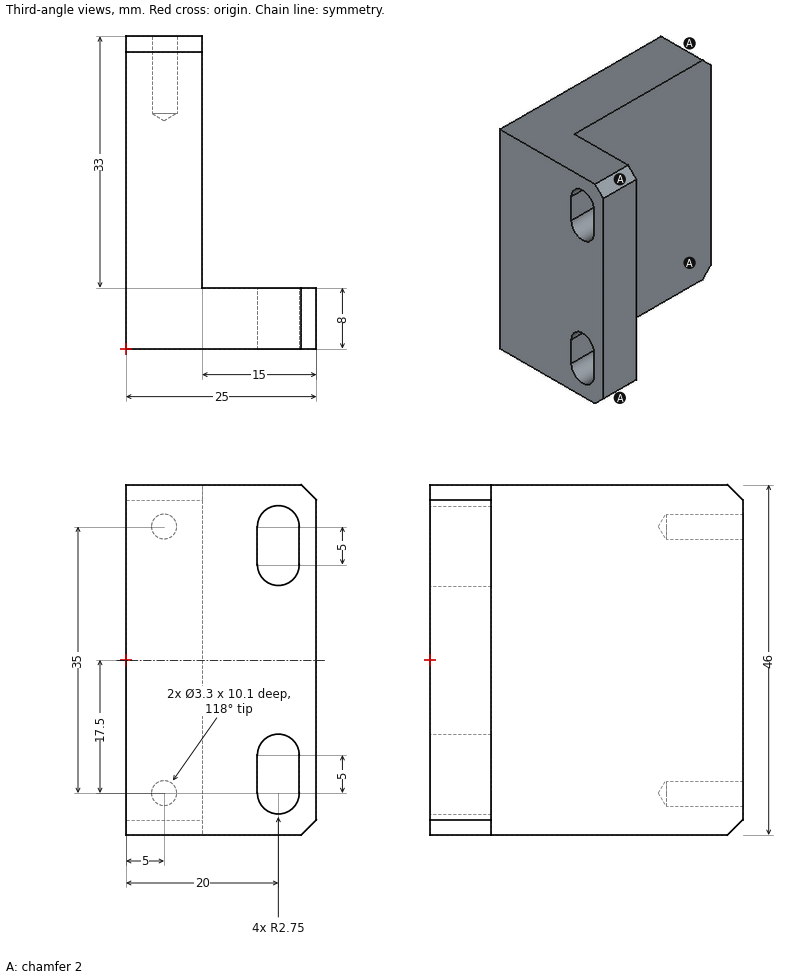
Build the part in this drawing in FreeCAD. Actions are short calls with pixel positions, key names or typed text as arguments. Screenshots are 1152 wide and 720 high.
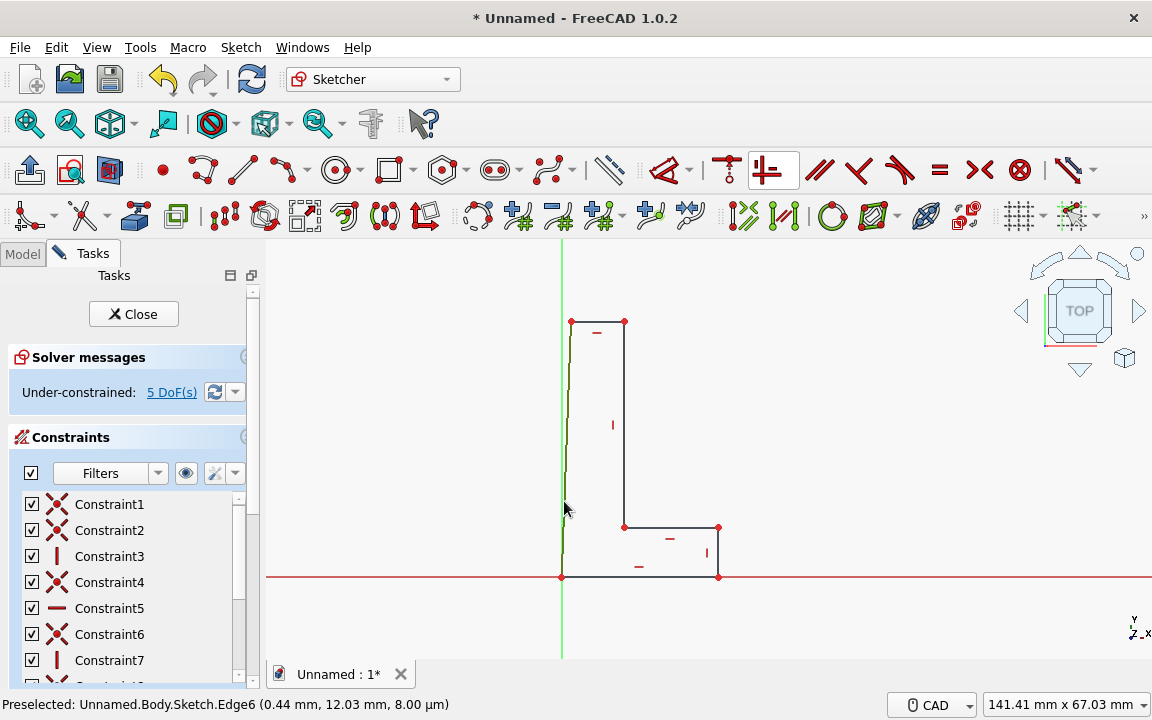
click(794, 170)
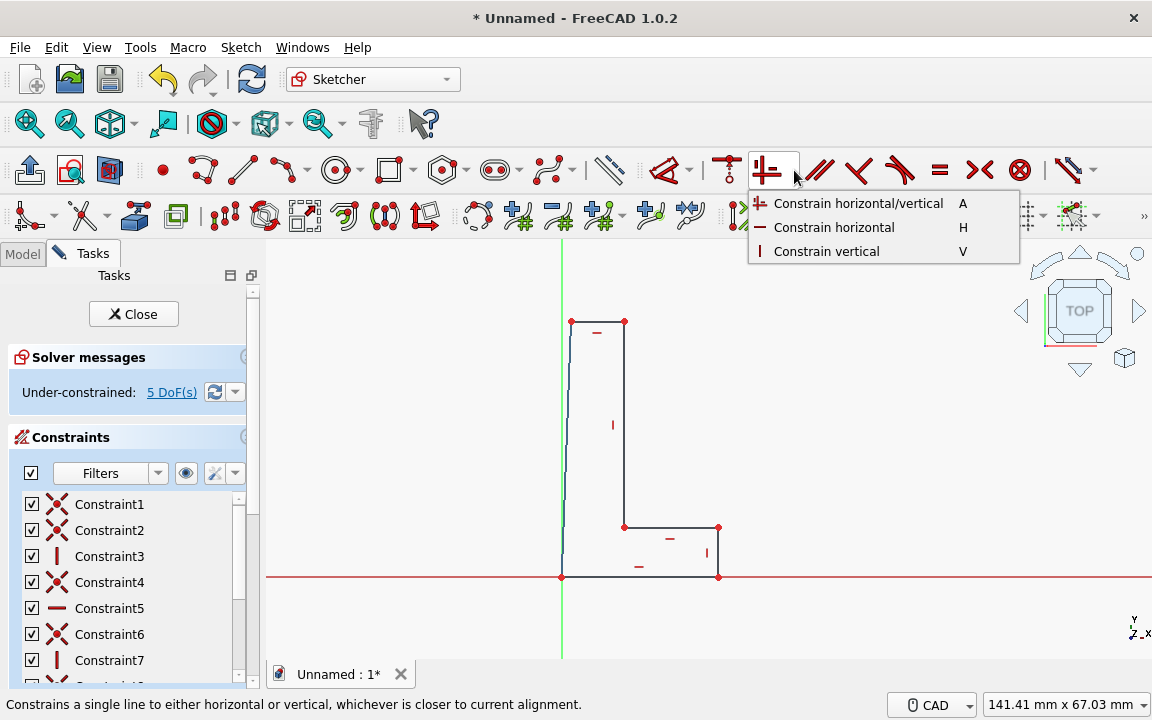
click(884, 251)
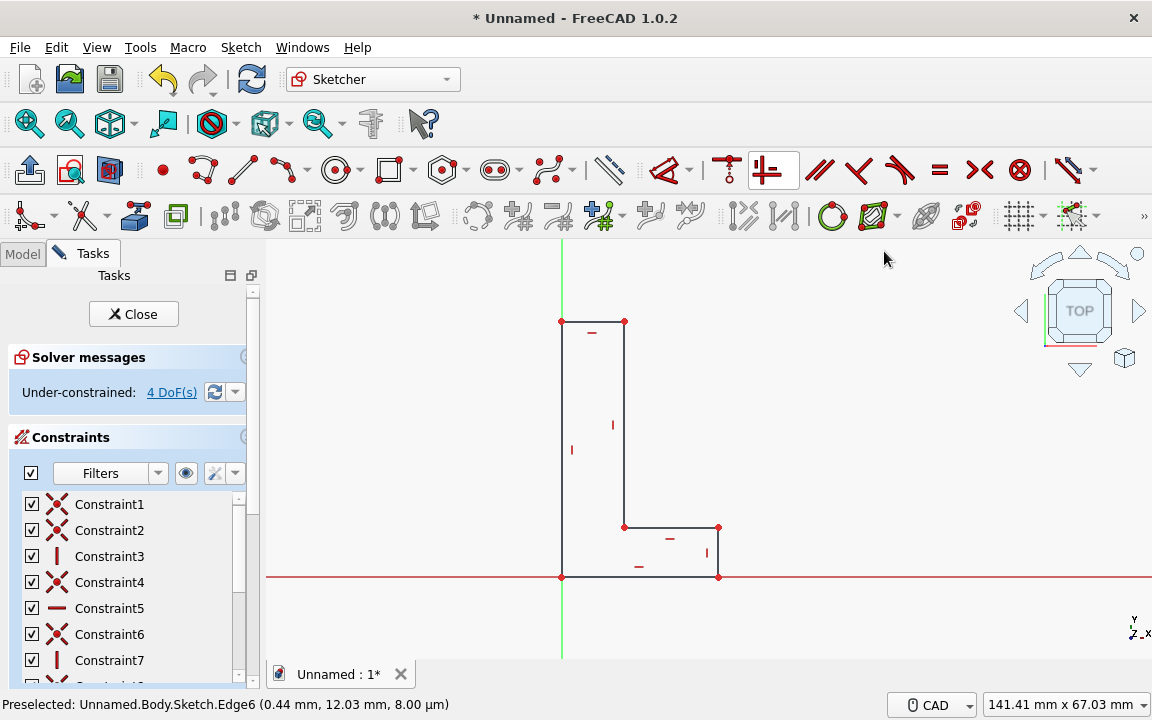
click(718, 563)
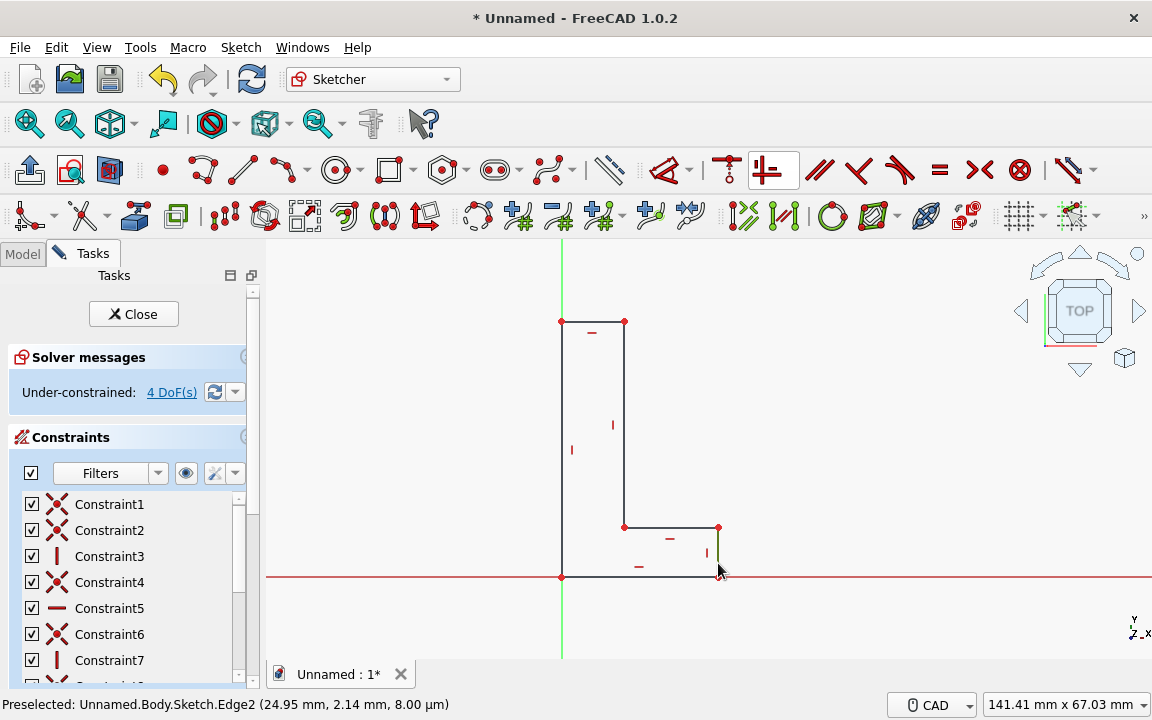
key(i)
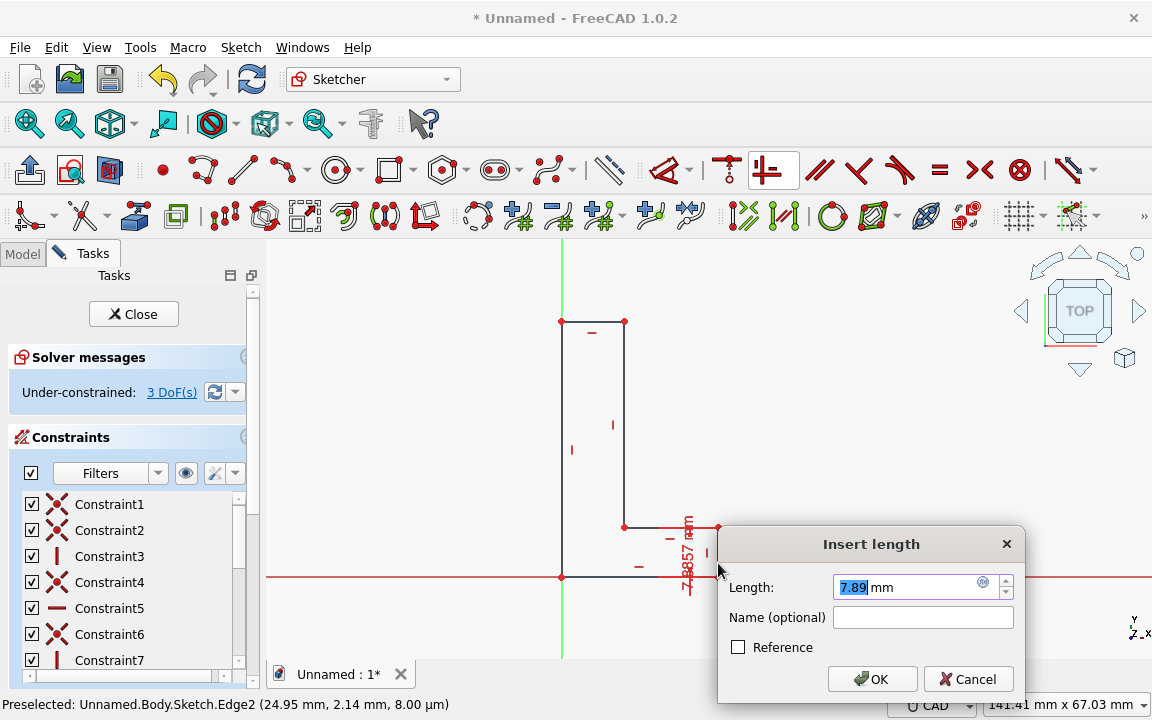
text(8)
key(Return)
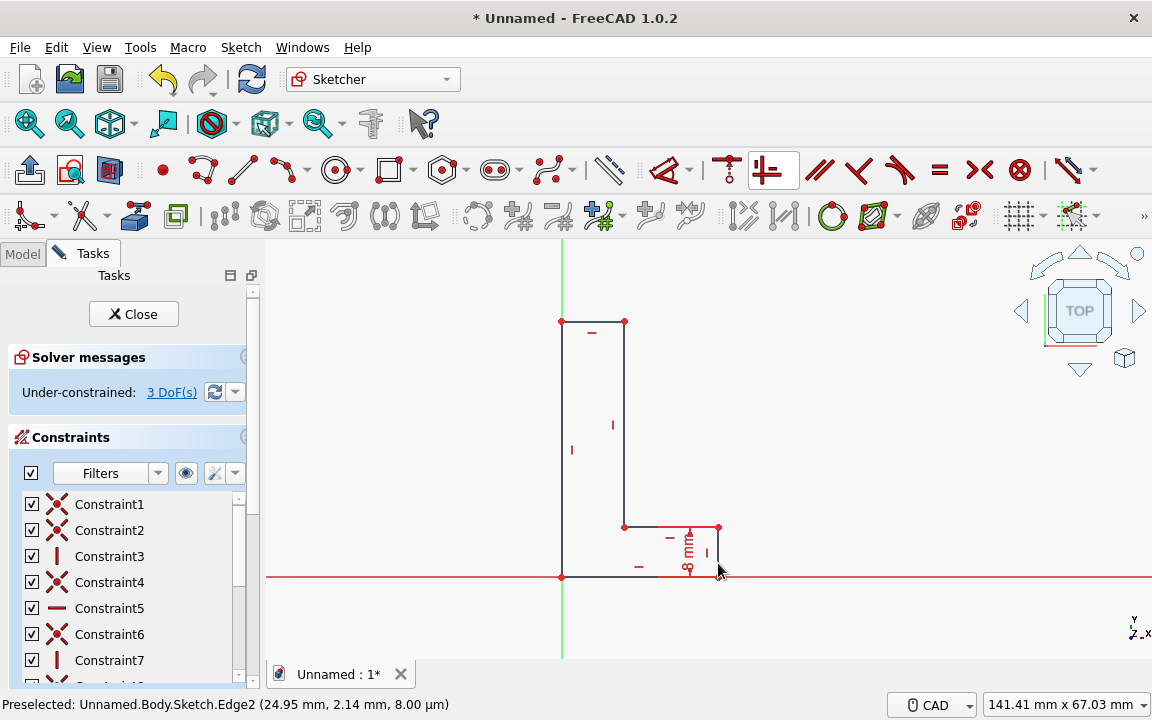
click(609, 577)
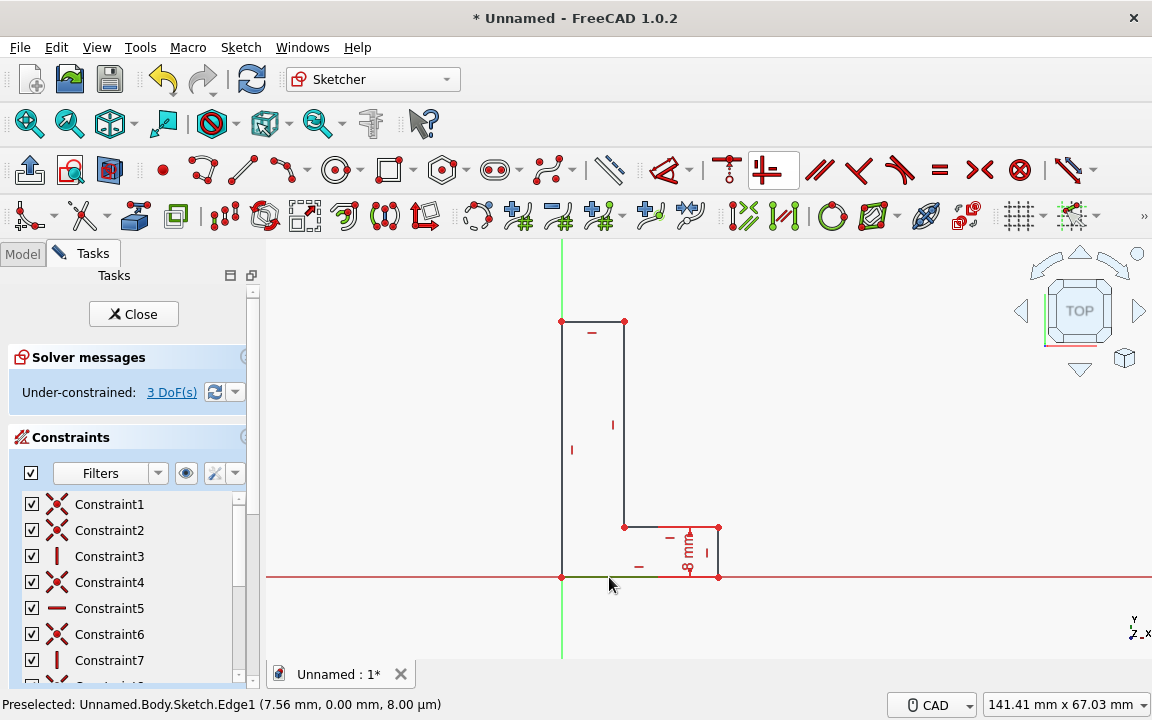
click(692, 170)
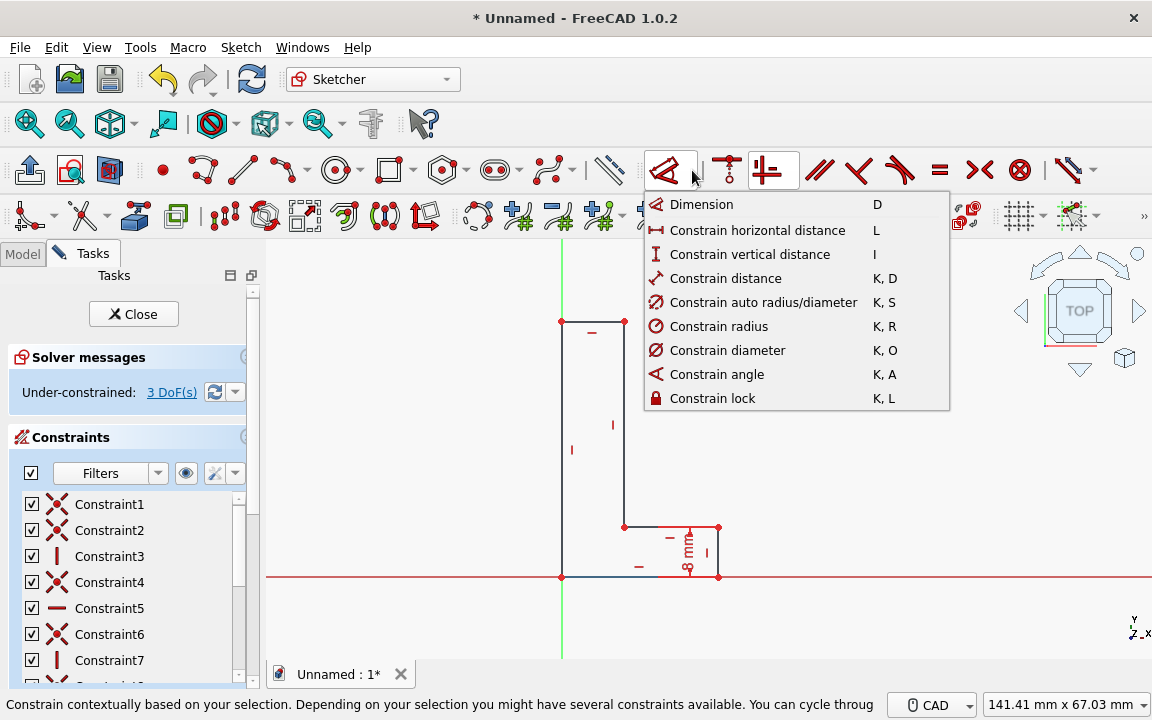
click(797, 230)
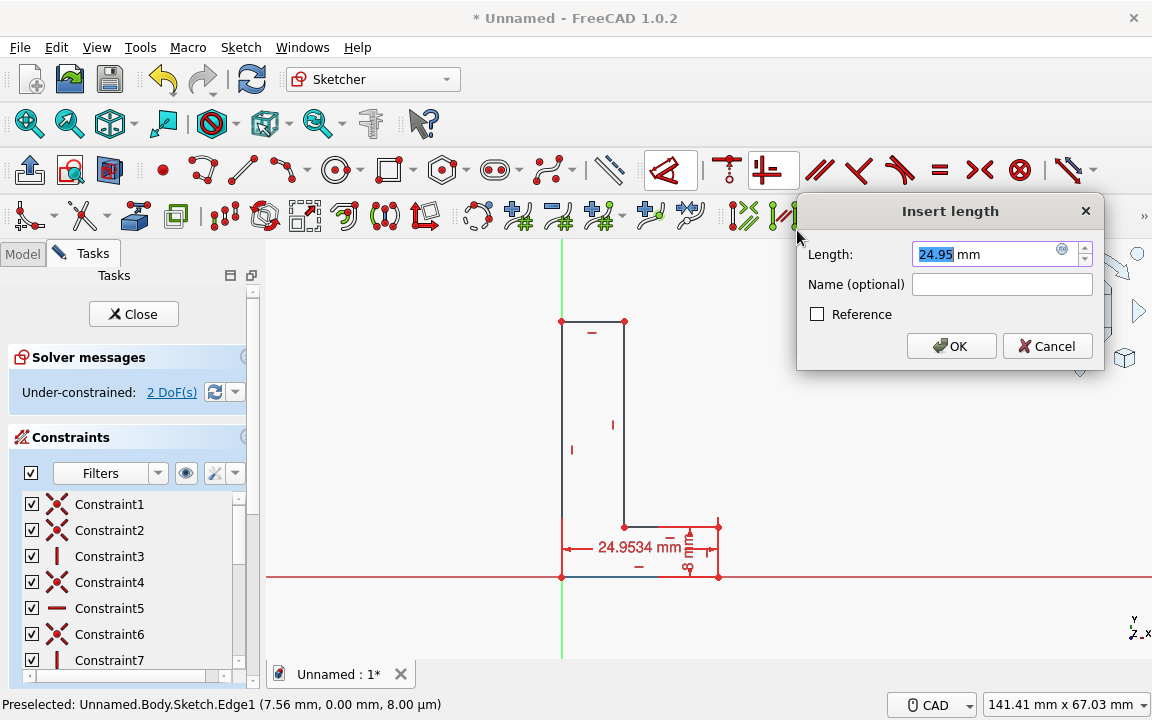
text(25)
key(Return)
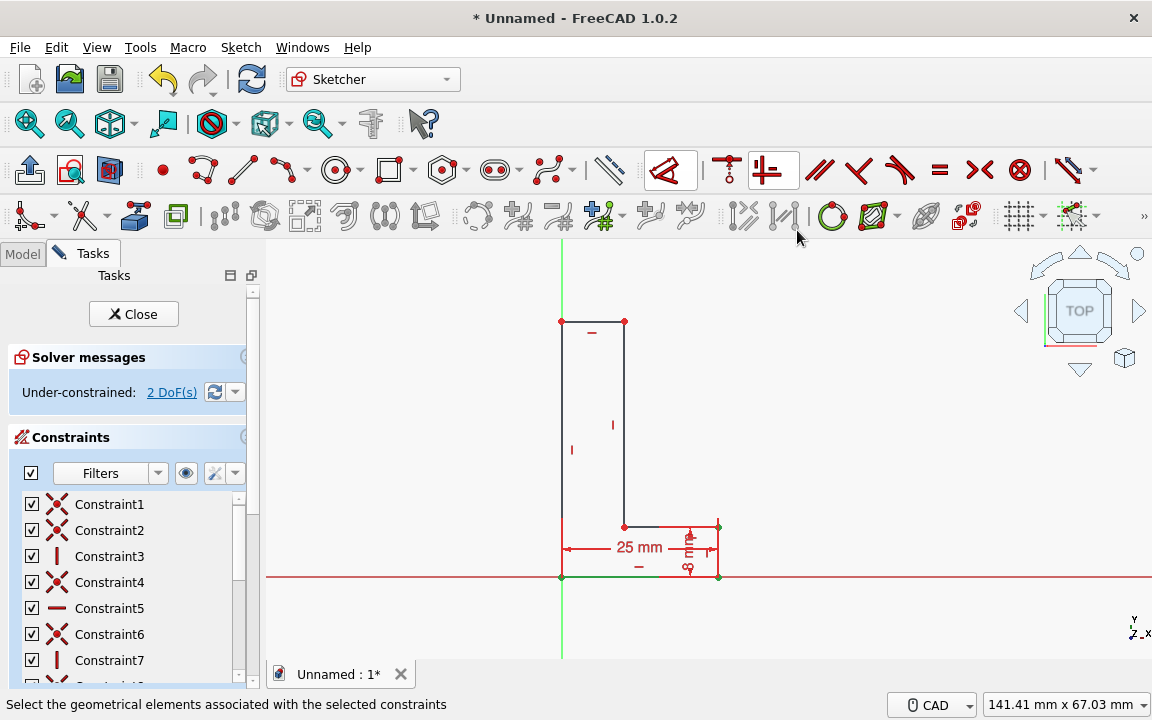
click(690, 527)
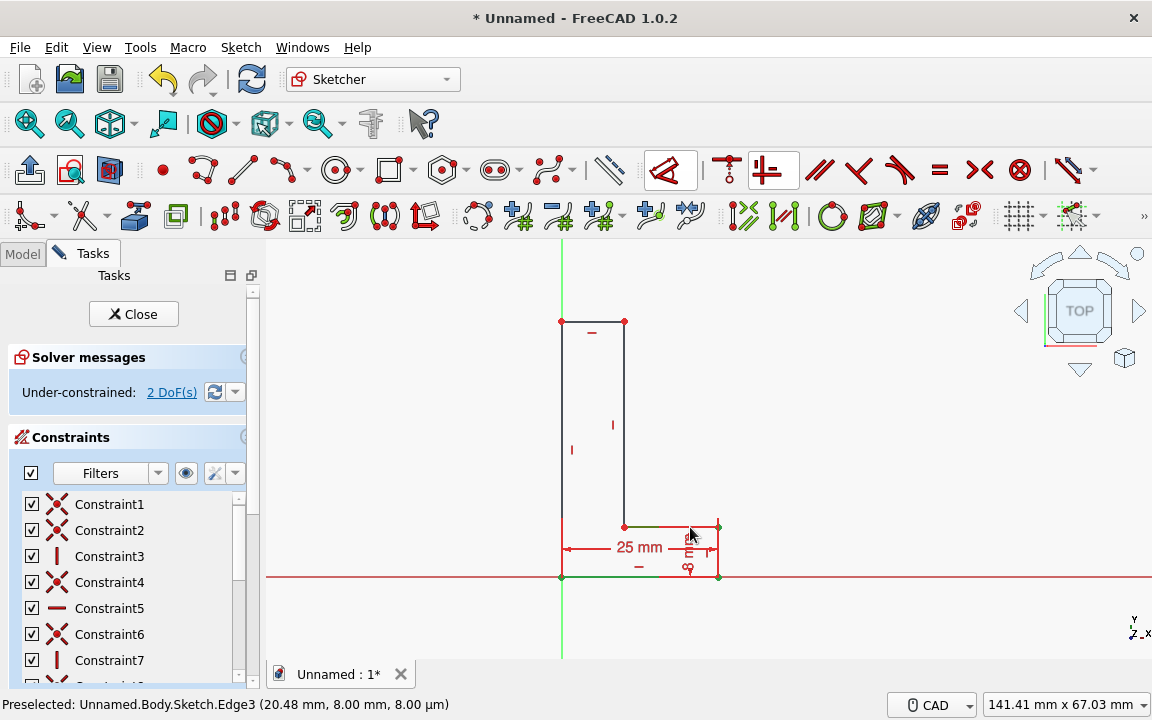
key(l)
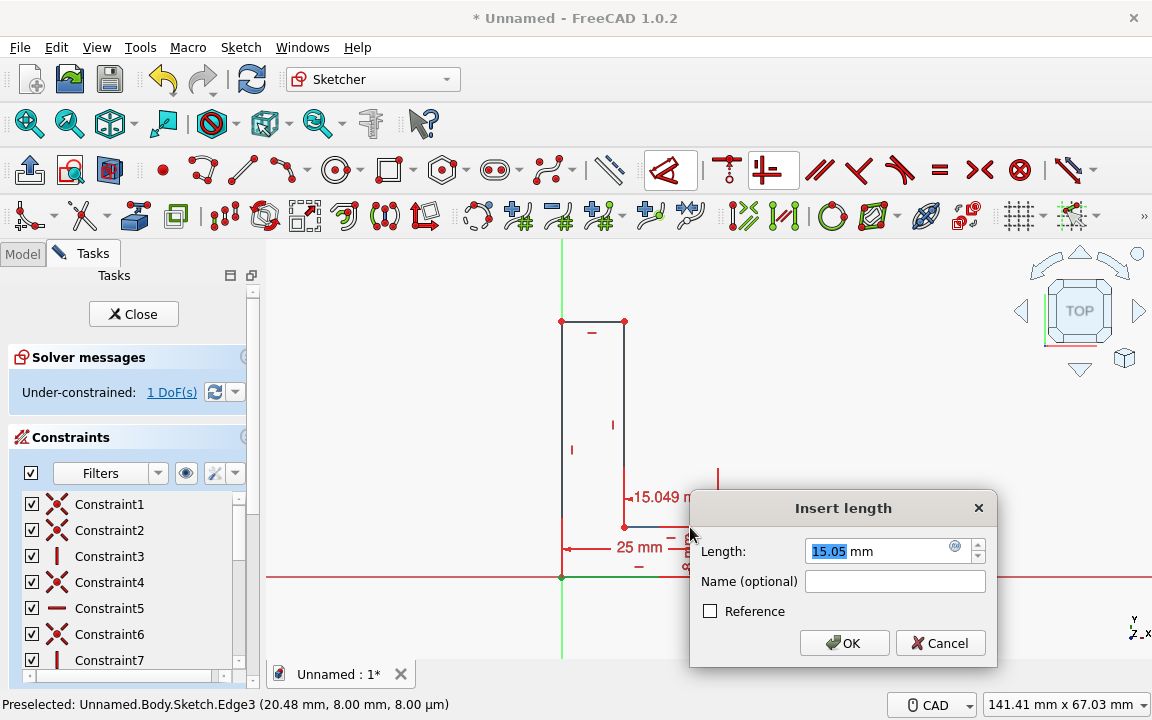
text(15)
key(Return)